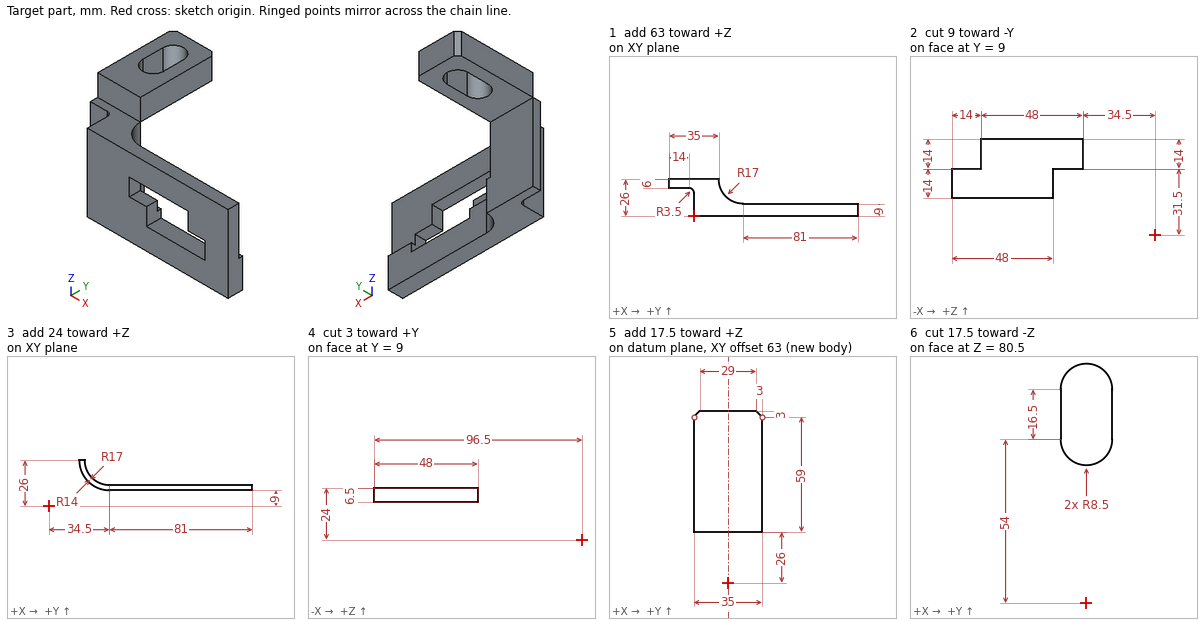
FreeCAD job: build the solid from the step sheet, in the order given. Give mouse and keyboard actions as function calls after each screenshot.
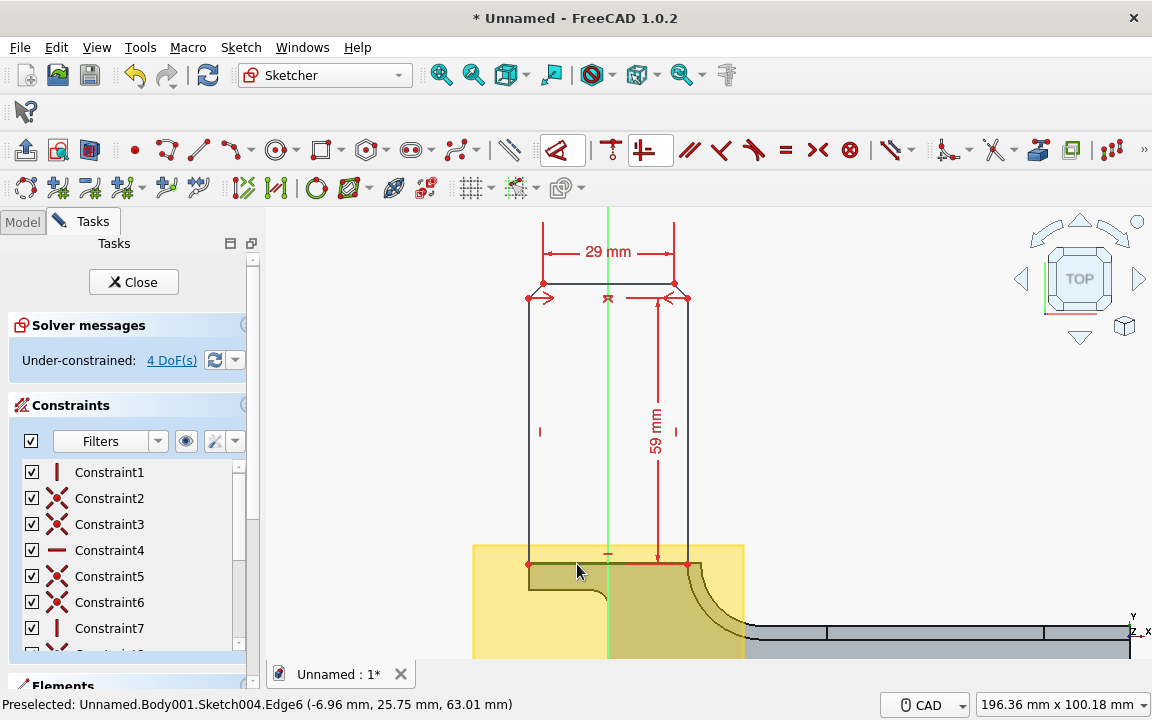
key(l)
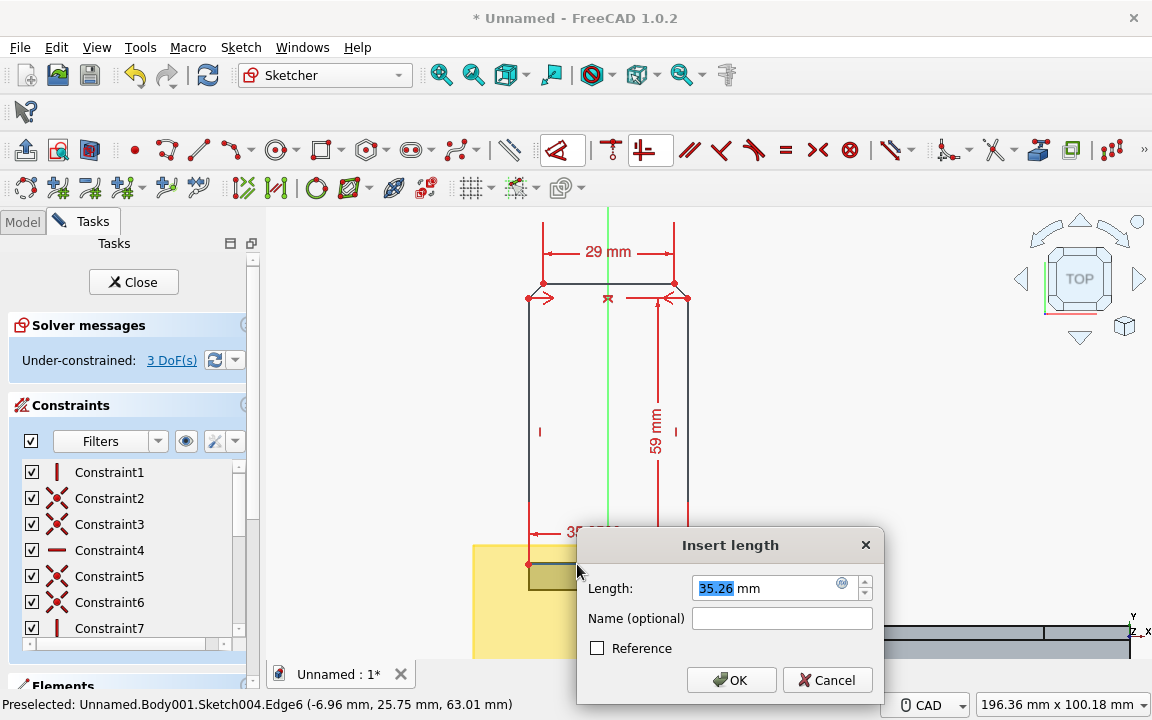
text(35)
key(Return)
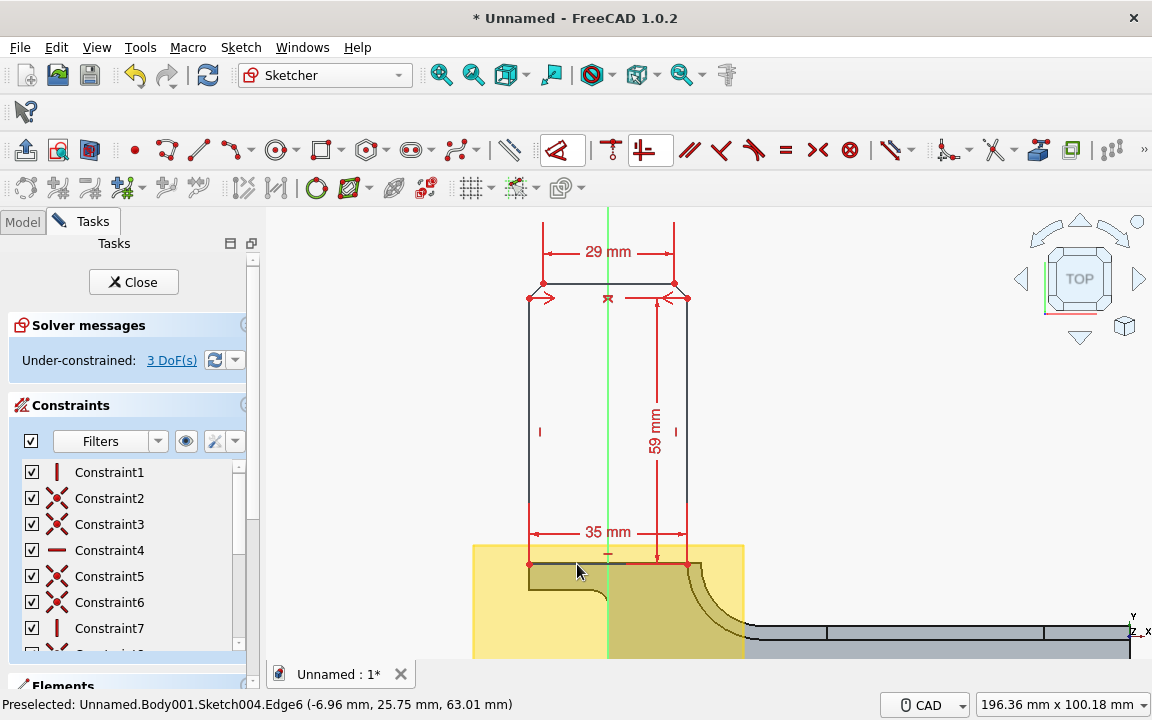
scroll(681, 291, up, 6)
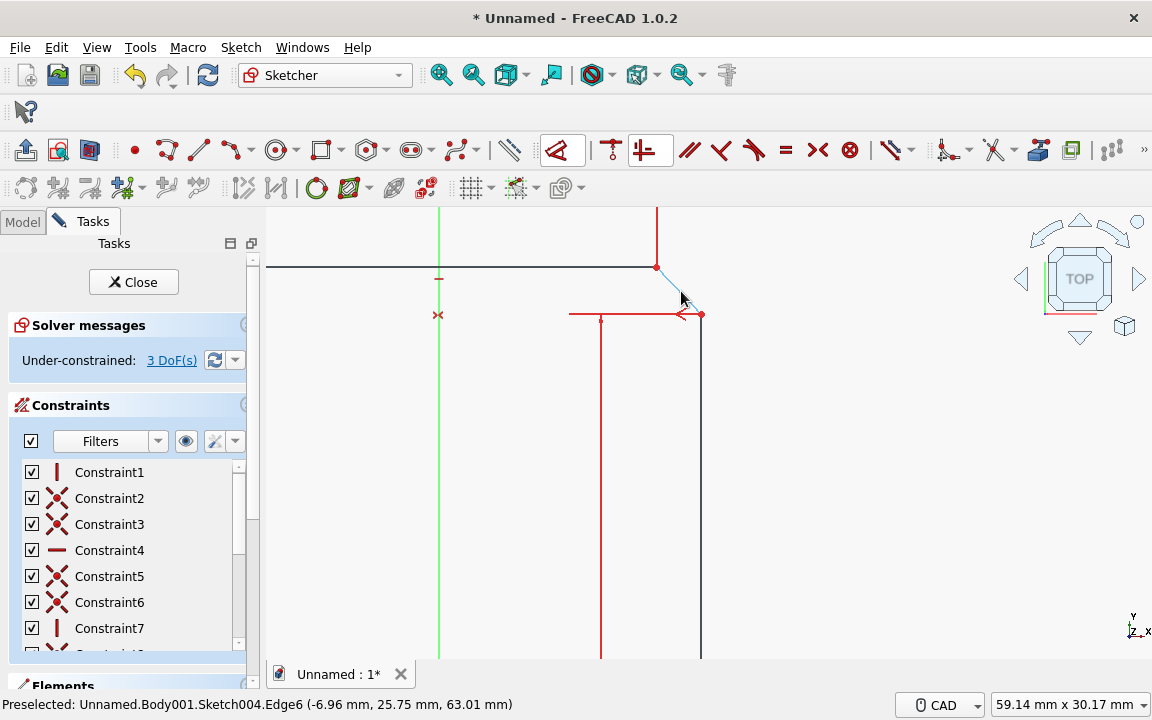
click(679, 291)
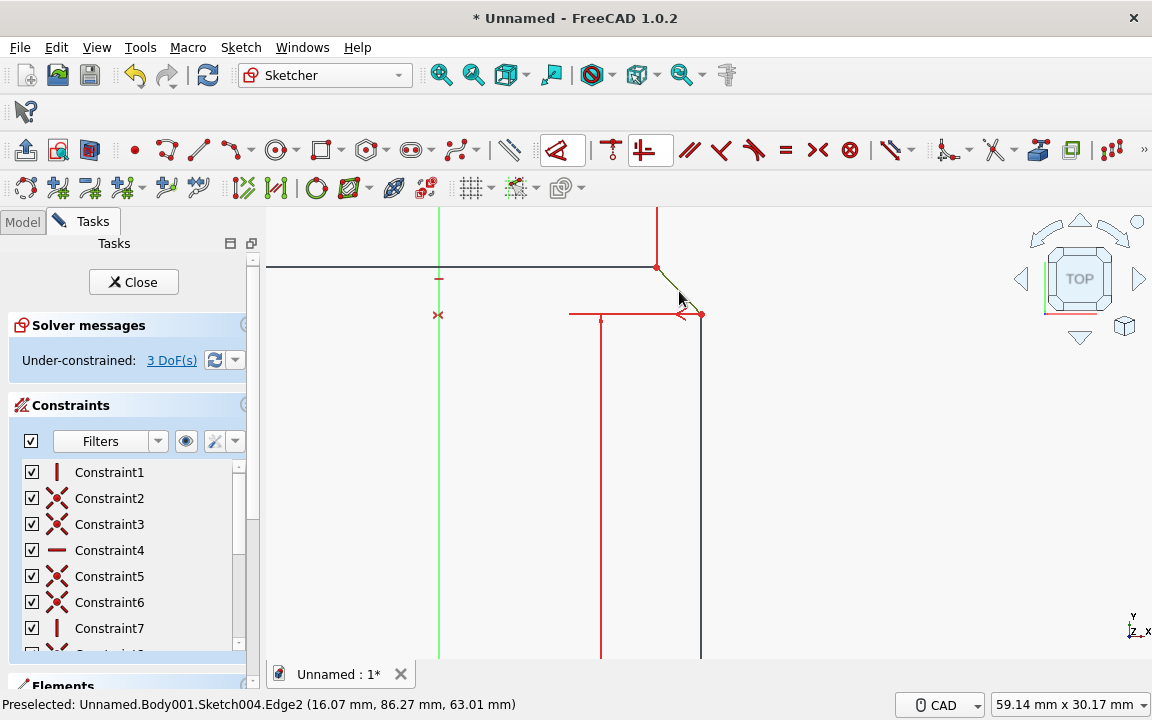
click(580, 150)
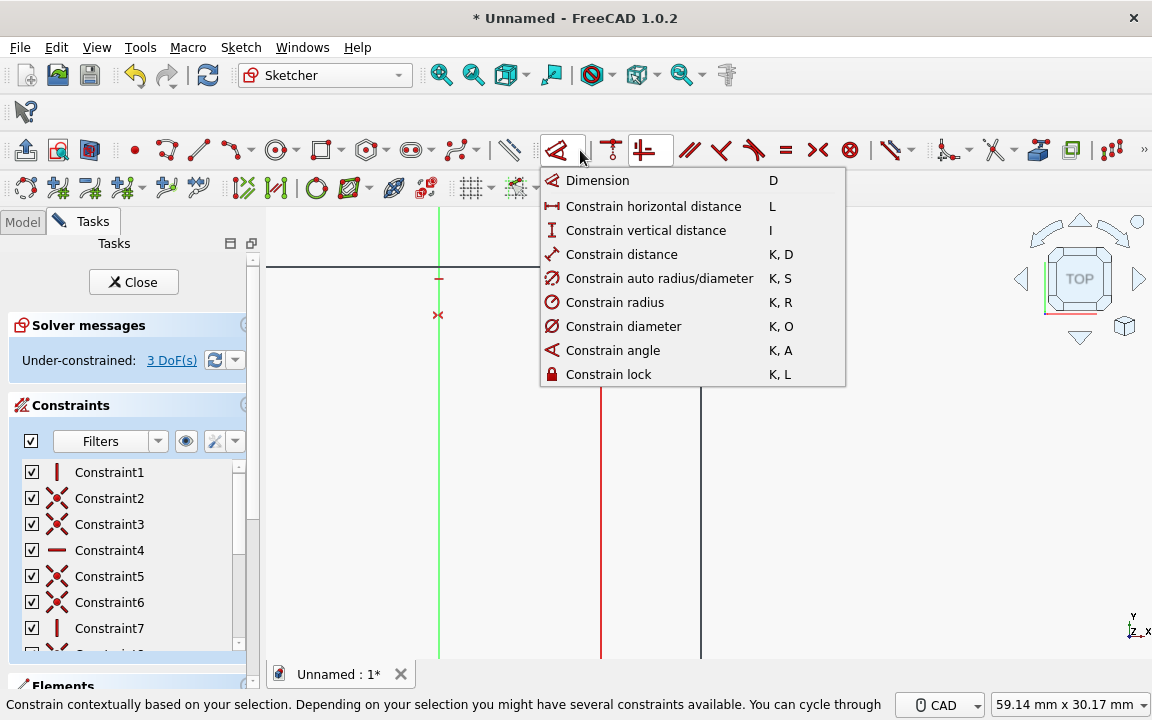
click(693, 206)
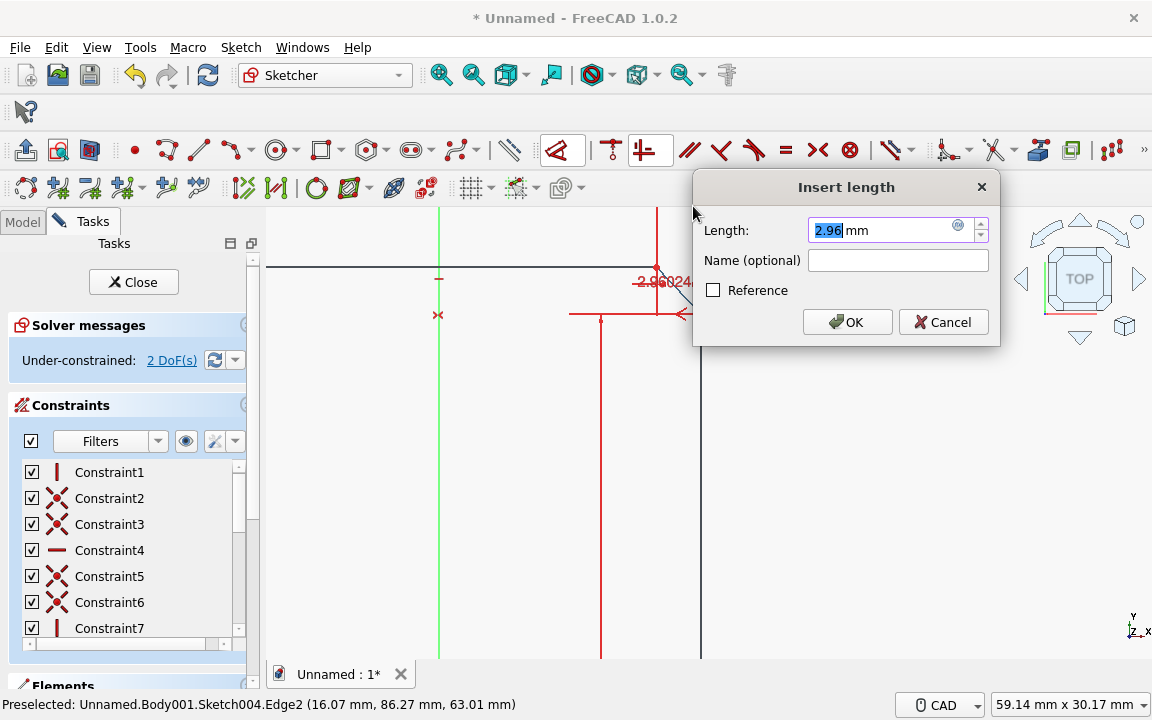
text(3)
key(Return)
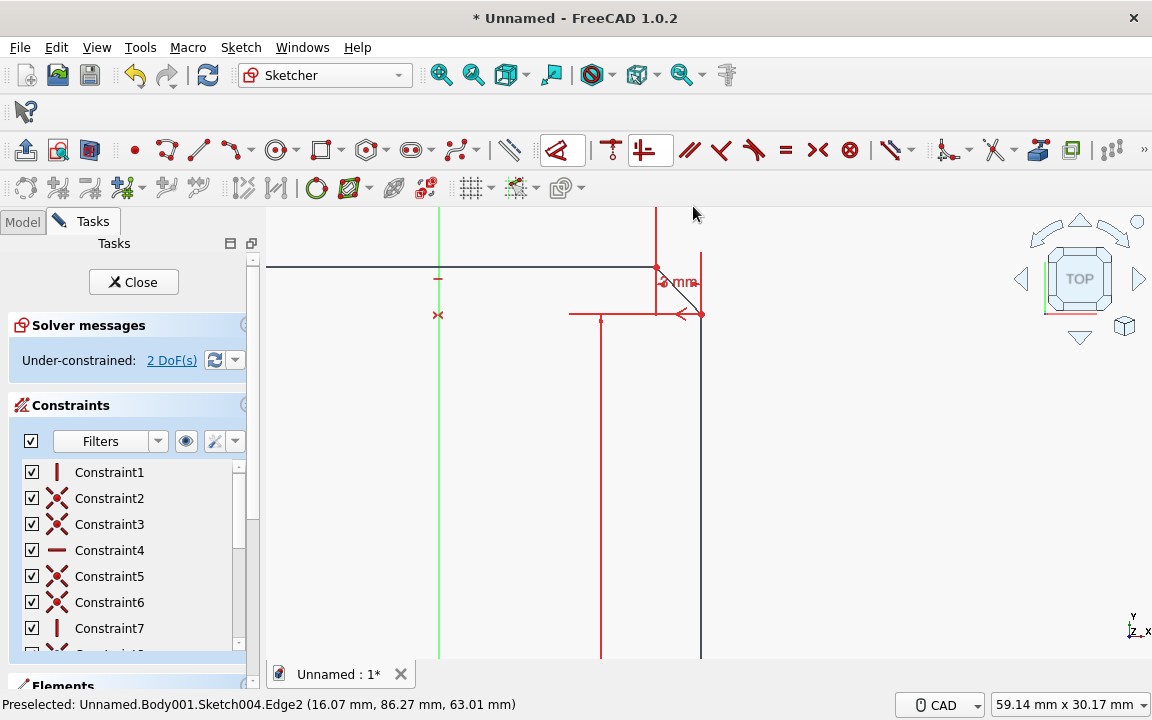
click(688, 300)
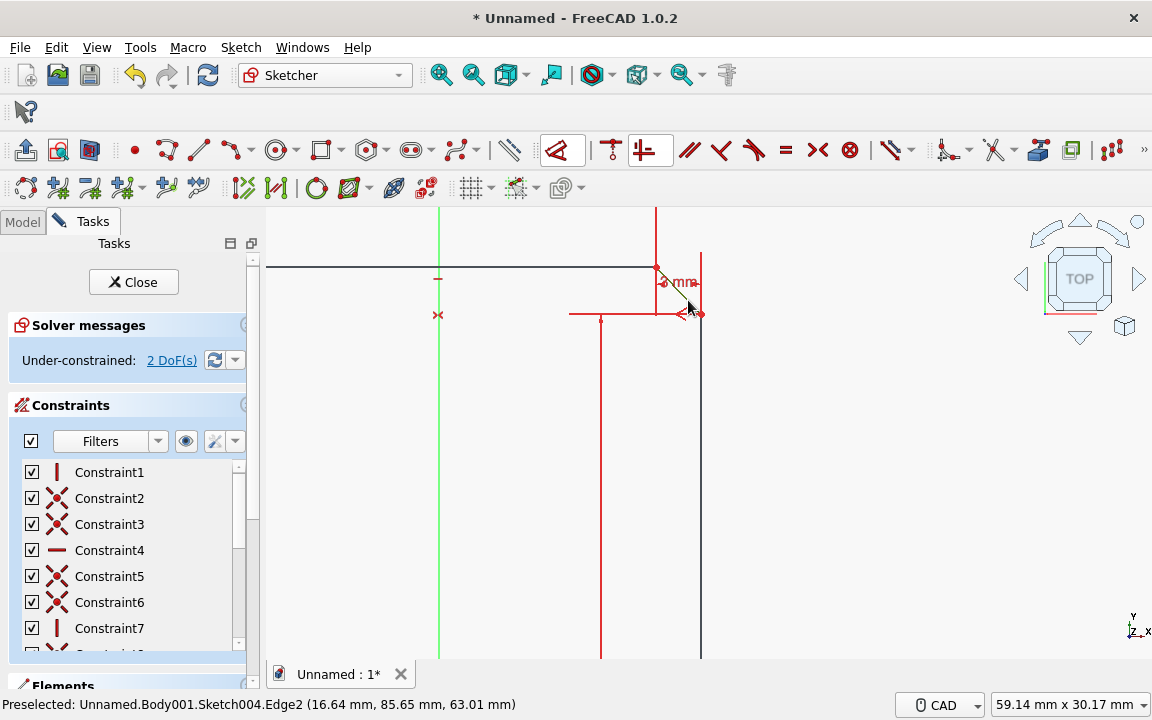
key(i)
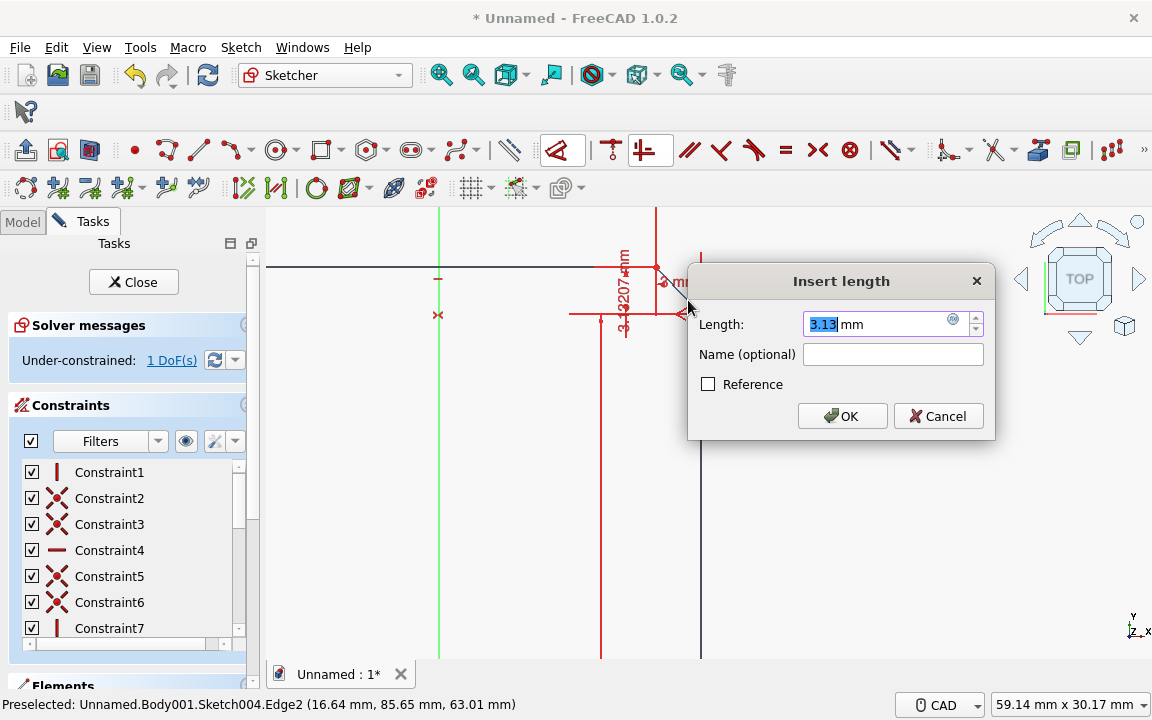
text(3)
key(Return)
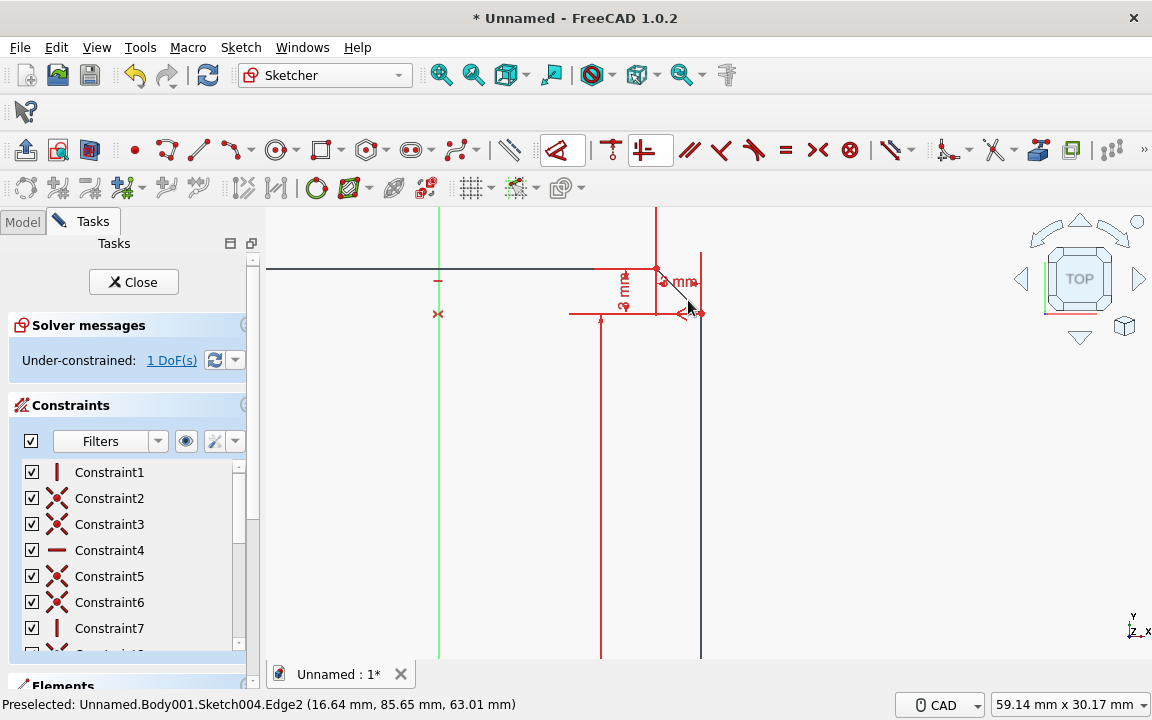
scroll(692, 309, down, 8)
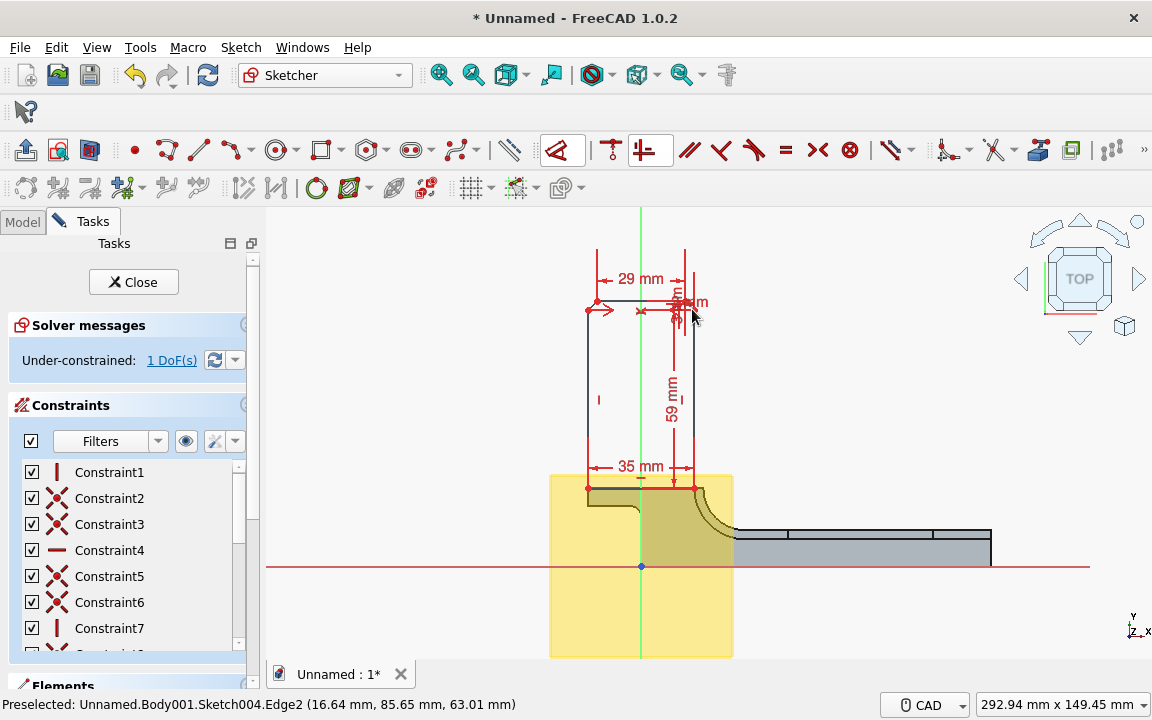
click(694, 489)